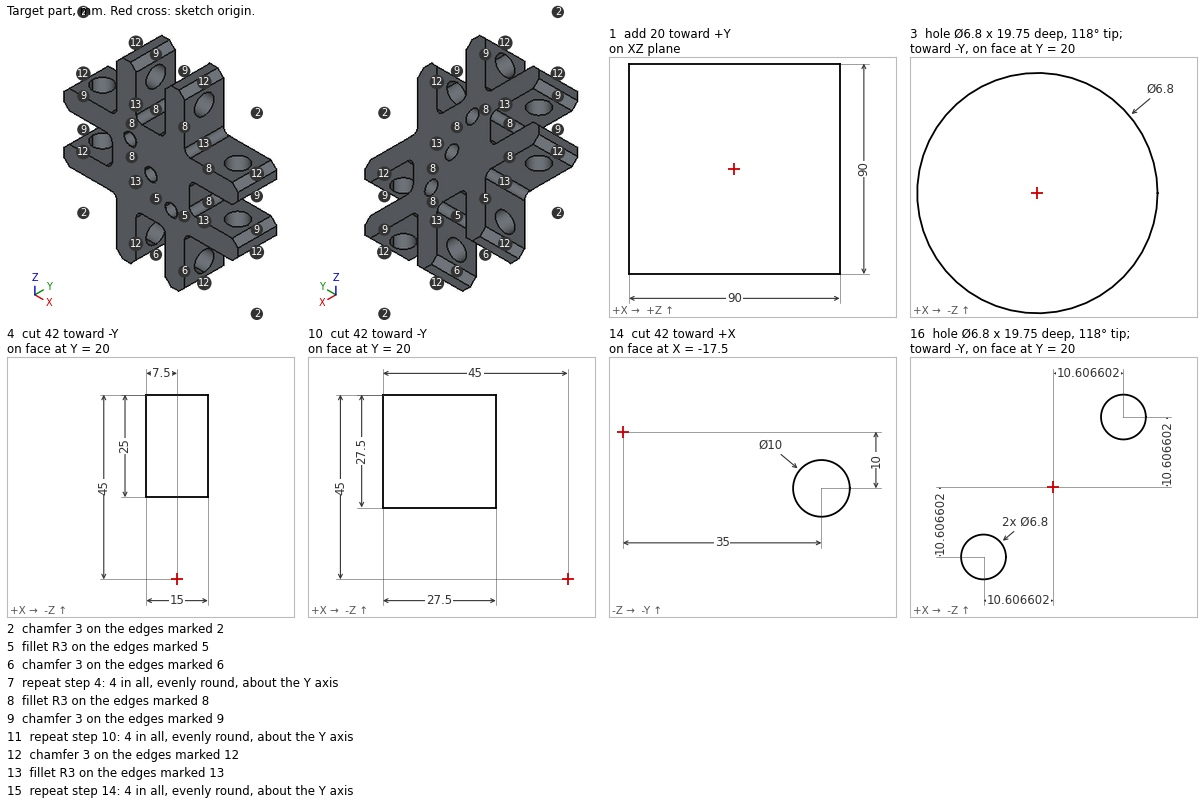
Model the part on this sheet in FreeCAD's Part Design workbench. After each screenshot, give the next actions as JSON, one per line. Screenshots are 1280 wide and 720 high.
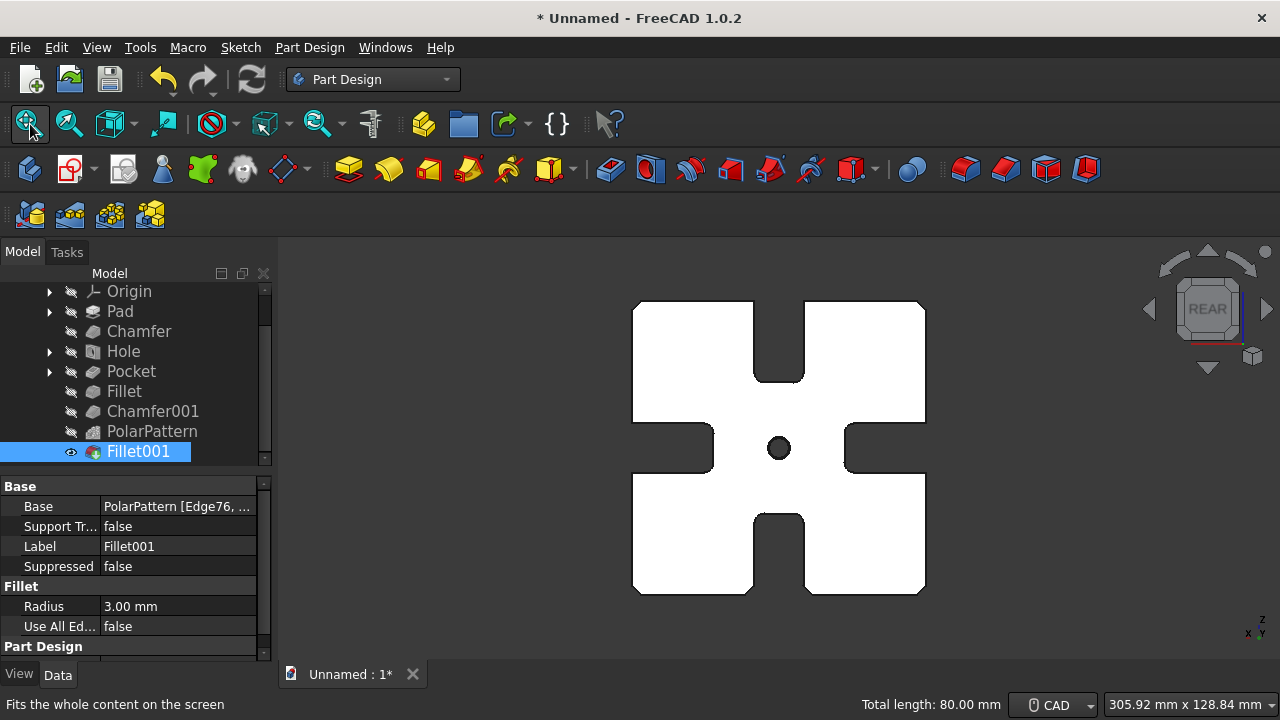
{"action": "key", "text": "6"}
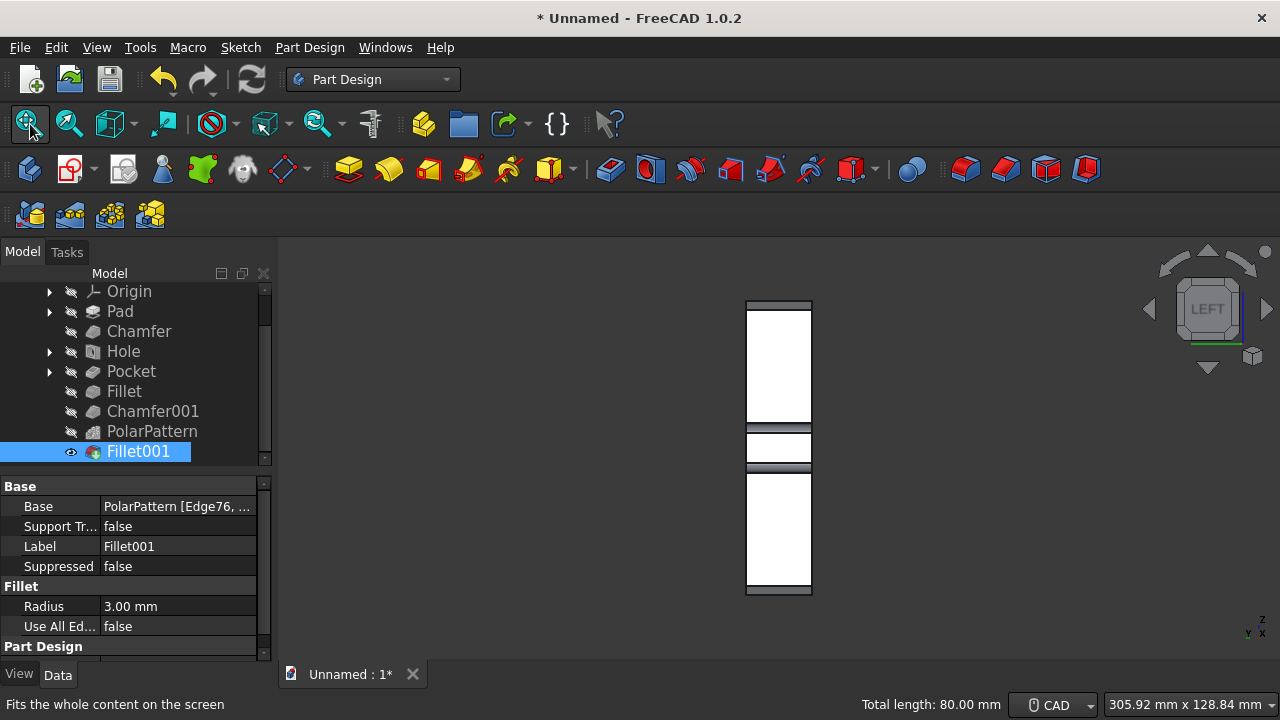
{"action": "left_click", "coordinate": [779, 472], "text": "ctrl"}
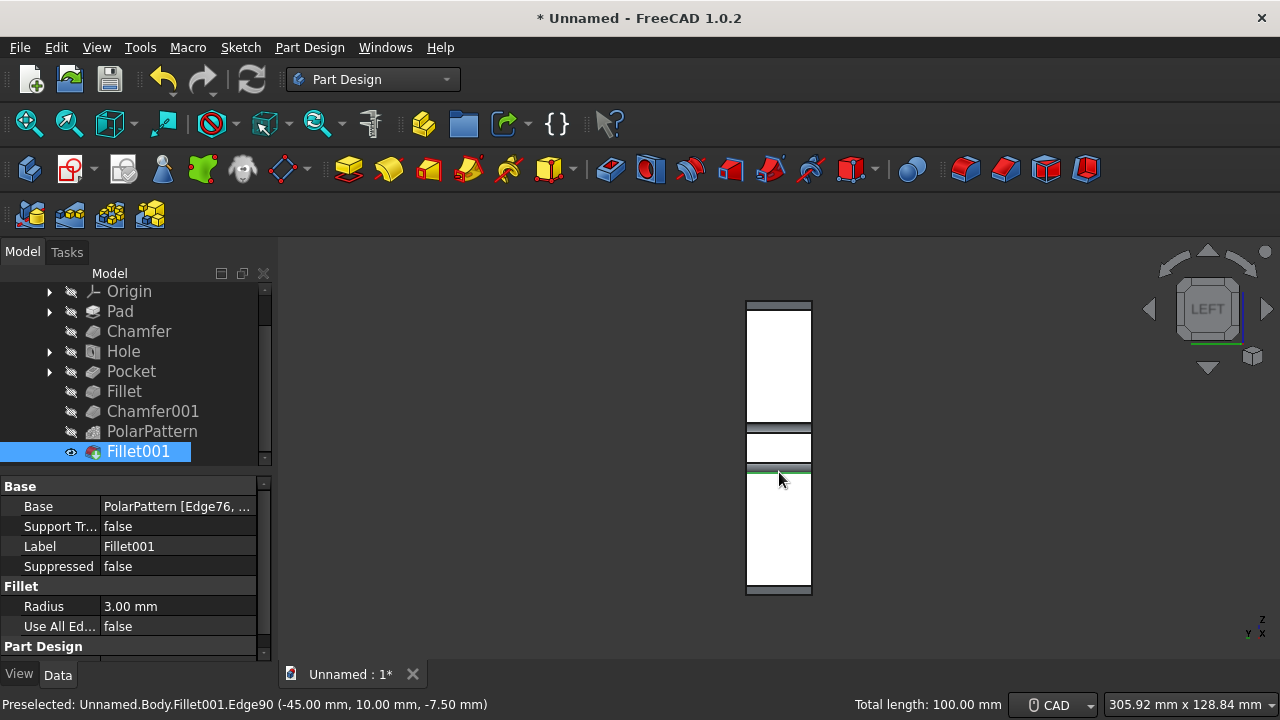
{"action": "left_click", "coordinate": [779, 422], "text": "ctrl"}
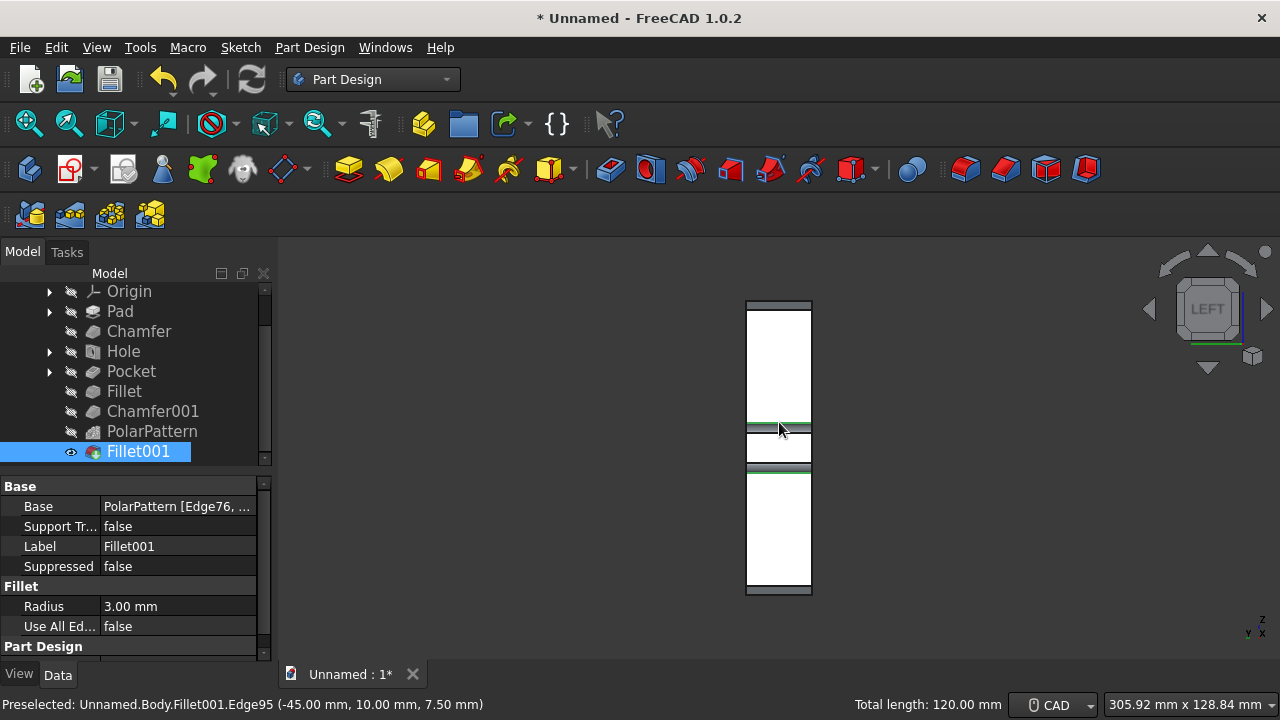
{"action": "left_click", "coordinate": [1006, 170]}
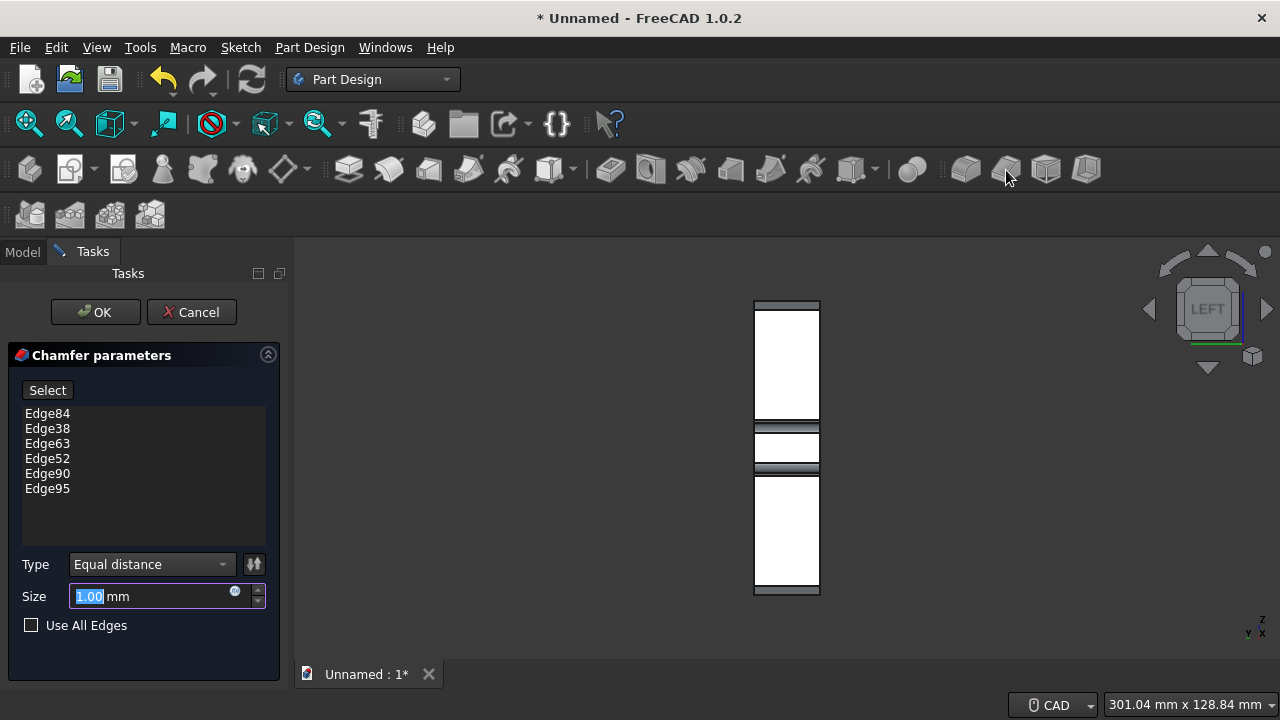
{"action": "type", "text": "3"}
{"action": "key", "text": "Tab"}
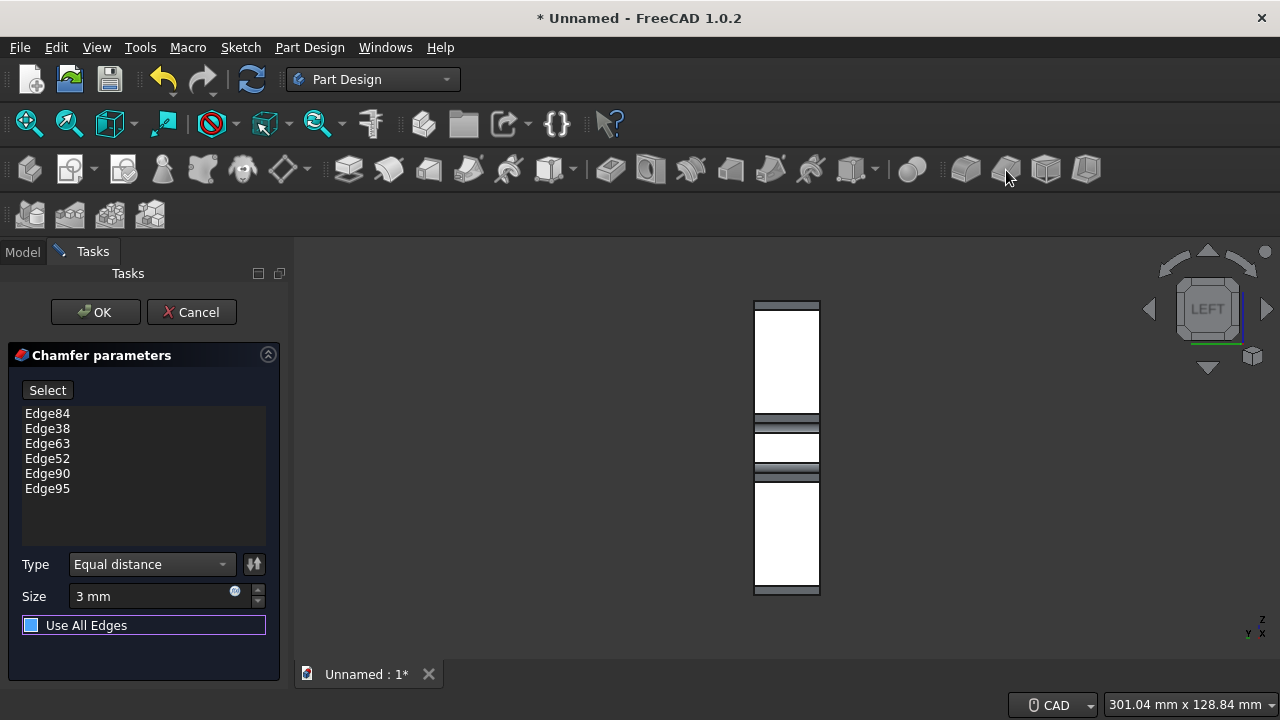
{"action": "left_click", "coordinate": [96, 312]}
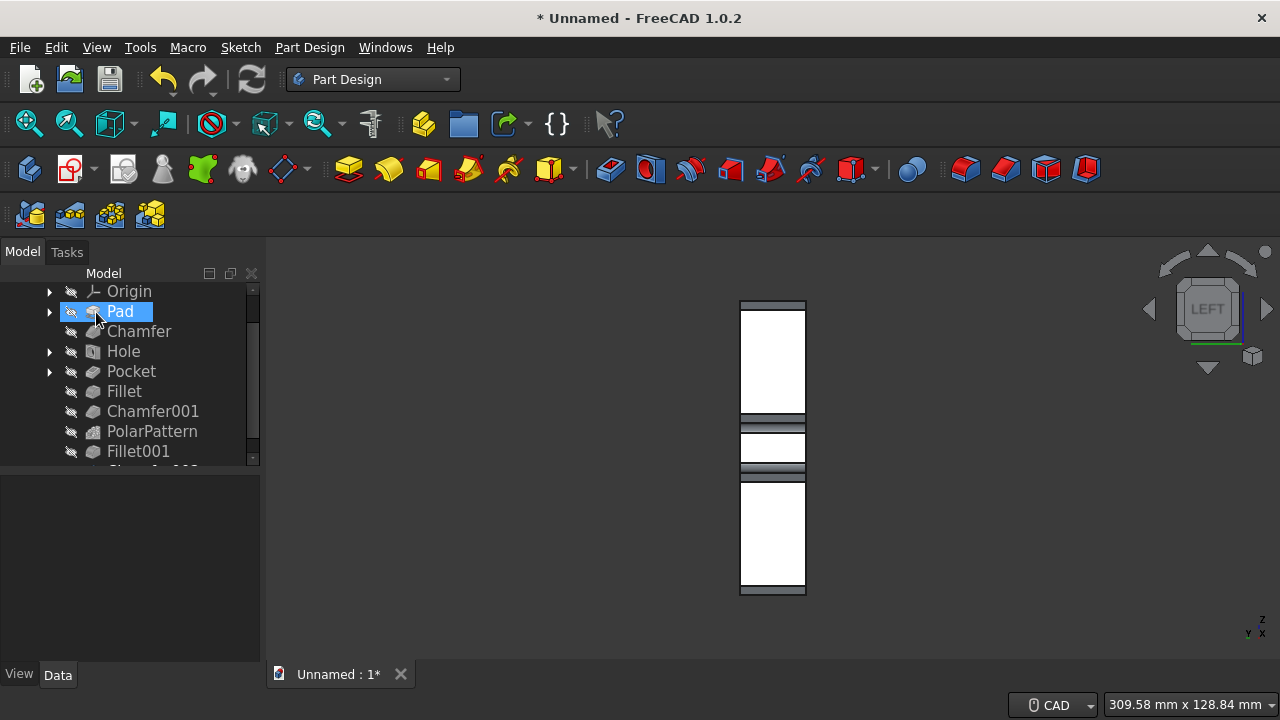
{"action": "key", "text": "4"}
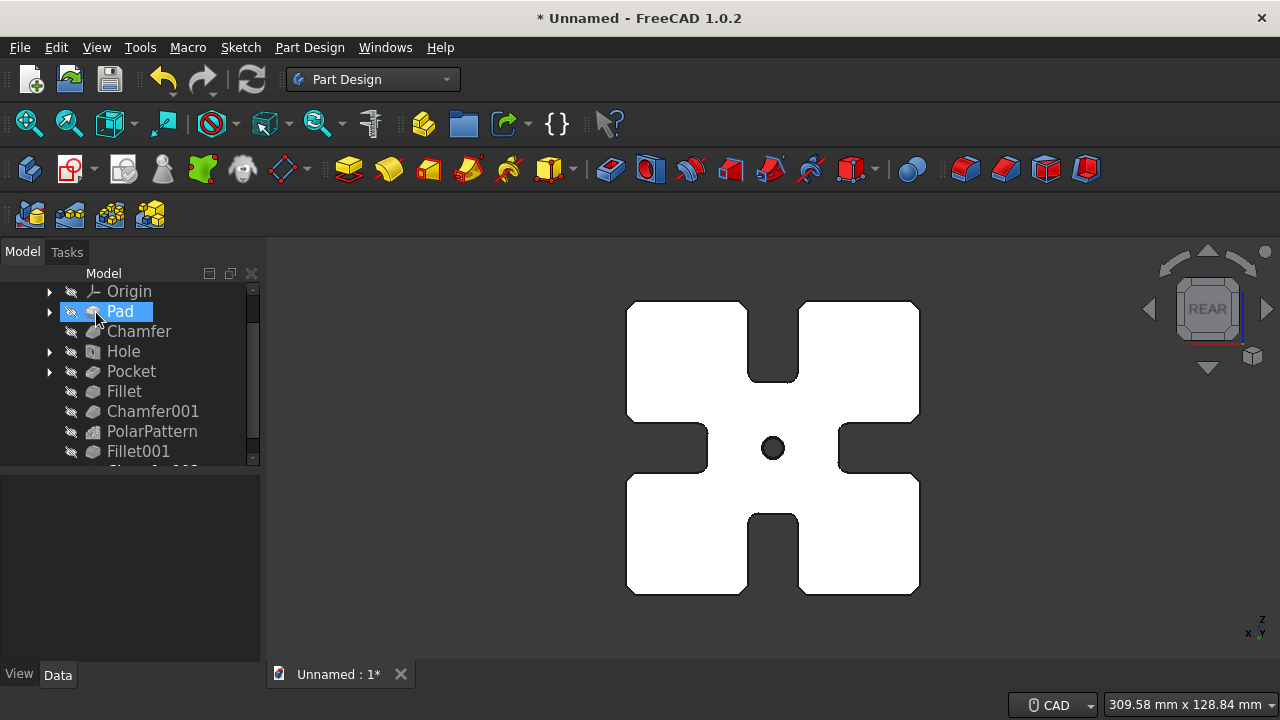
{"action": "left_click", "coordinate": [689, 531]}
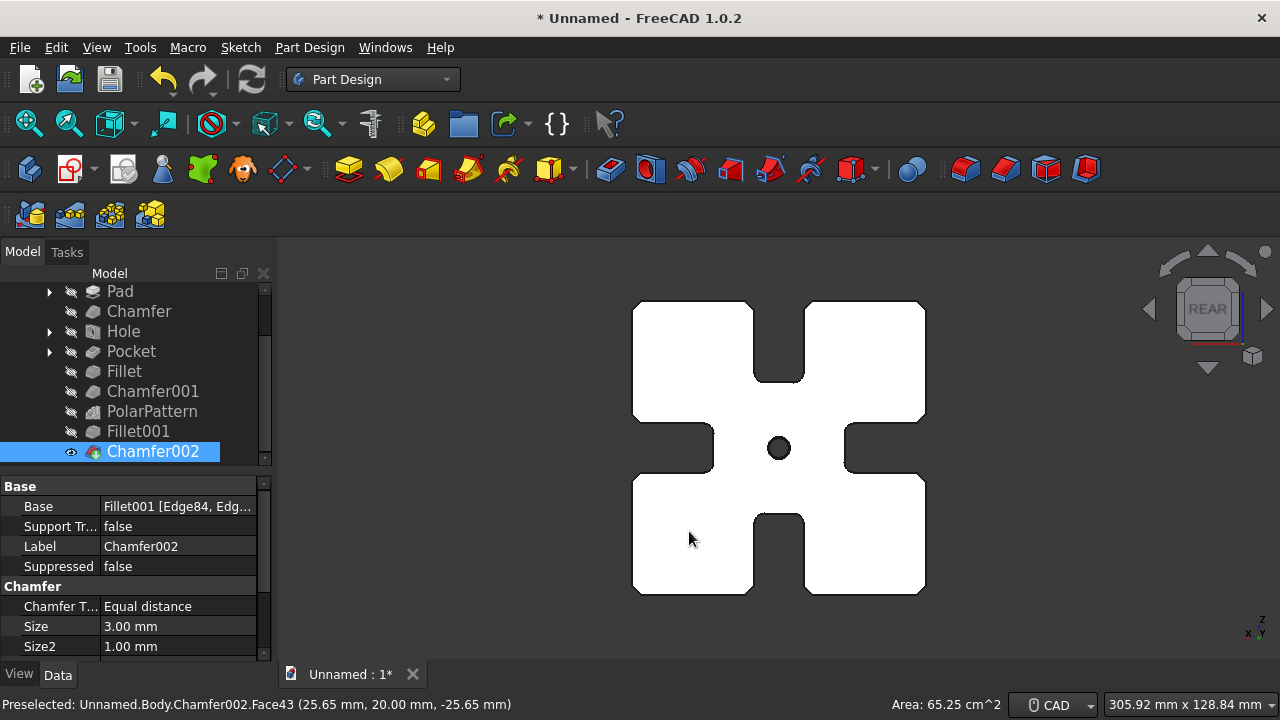
{"action": "left_click", "coordinate": [70, 170]}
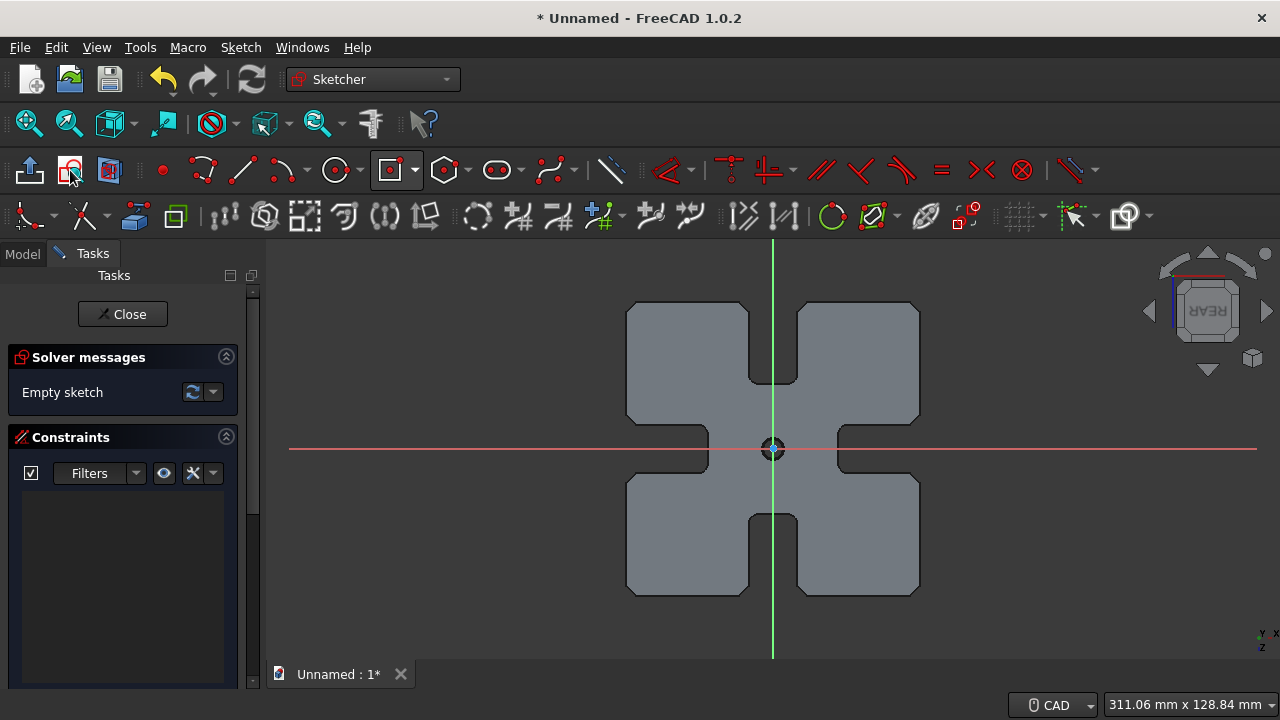
{"action": "scroll", "coordinate": [694, 286], "scroll_direction": "up", "scroll_amount": 3}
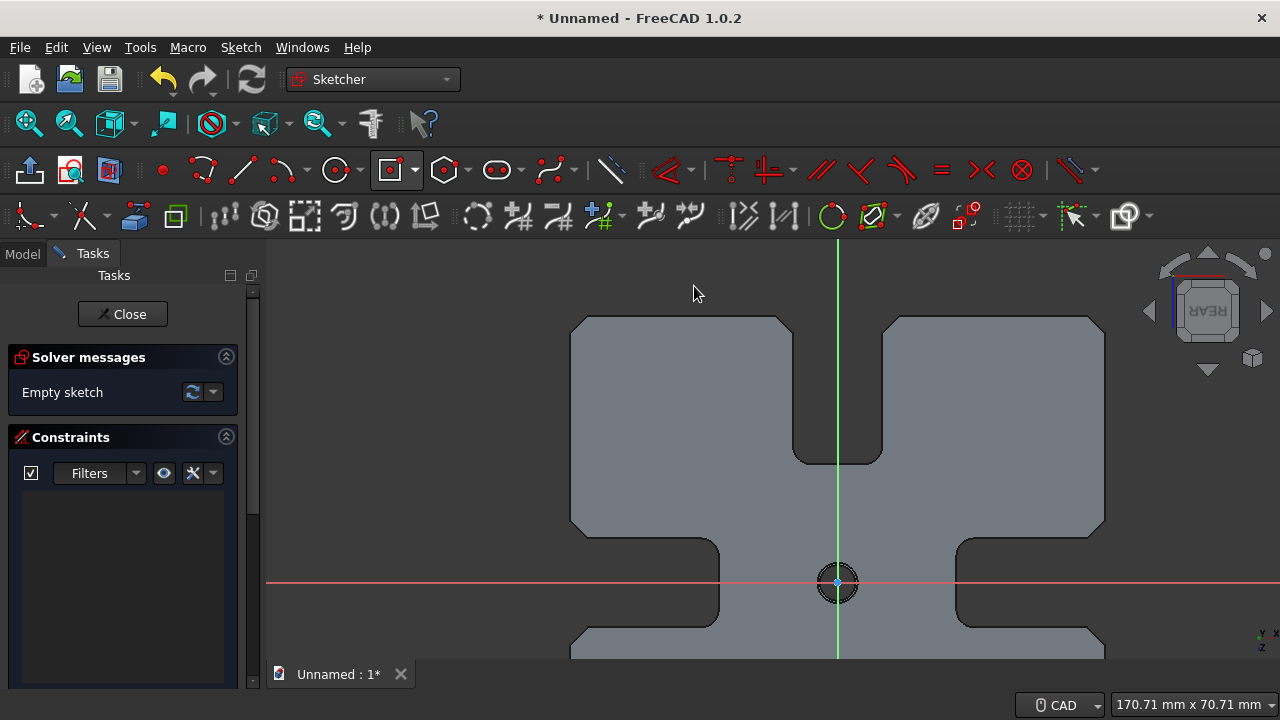
{"action": "left_click", "coordinate": [418, 170]}